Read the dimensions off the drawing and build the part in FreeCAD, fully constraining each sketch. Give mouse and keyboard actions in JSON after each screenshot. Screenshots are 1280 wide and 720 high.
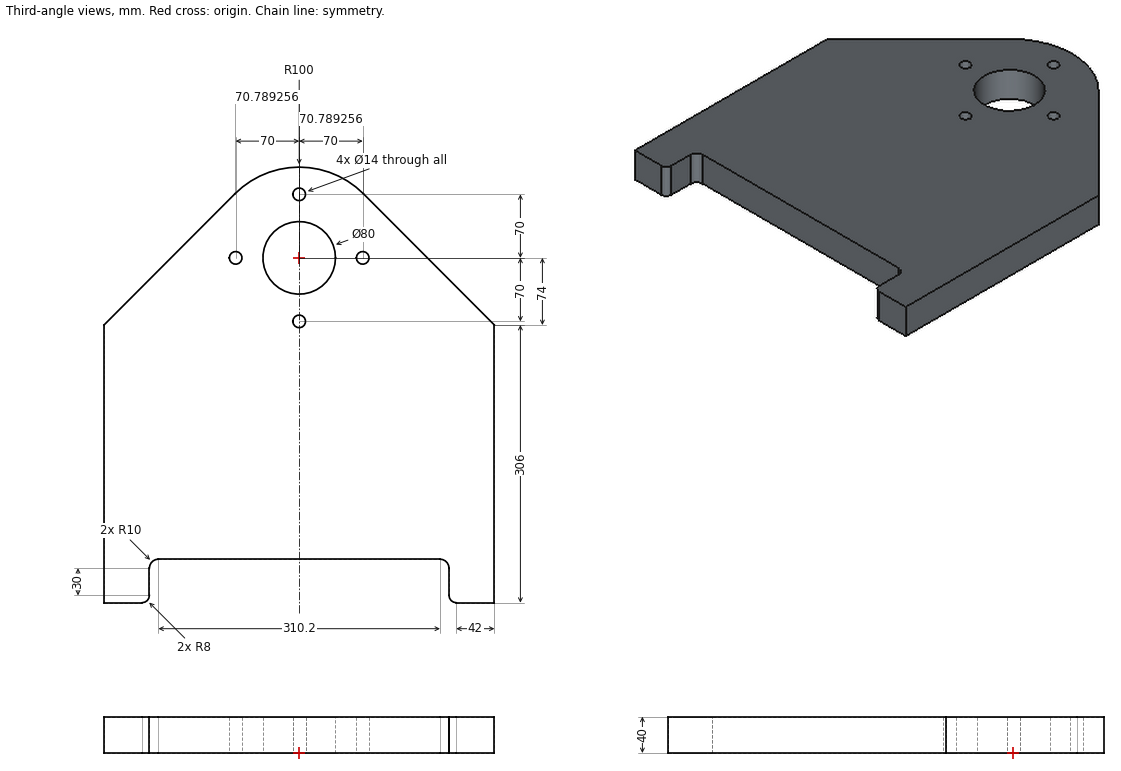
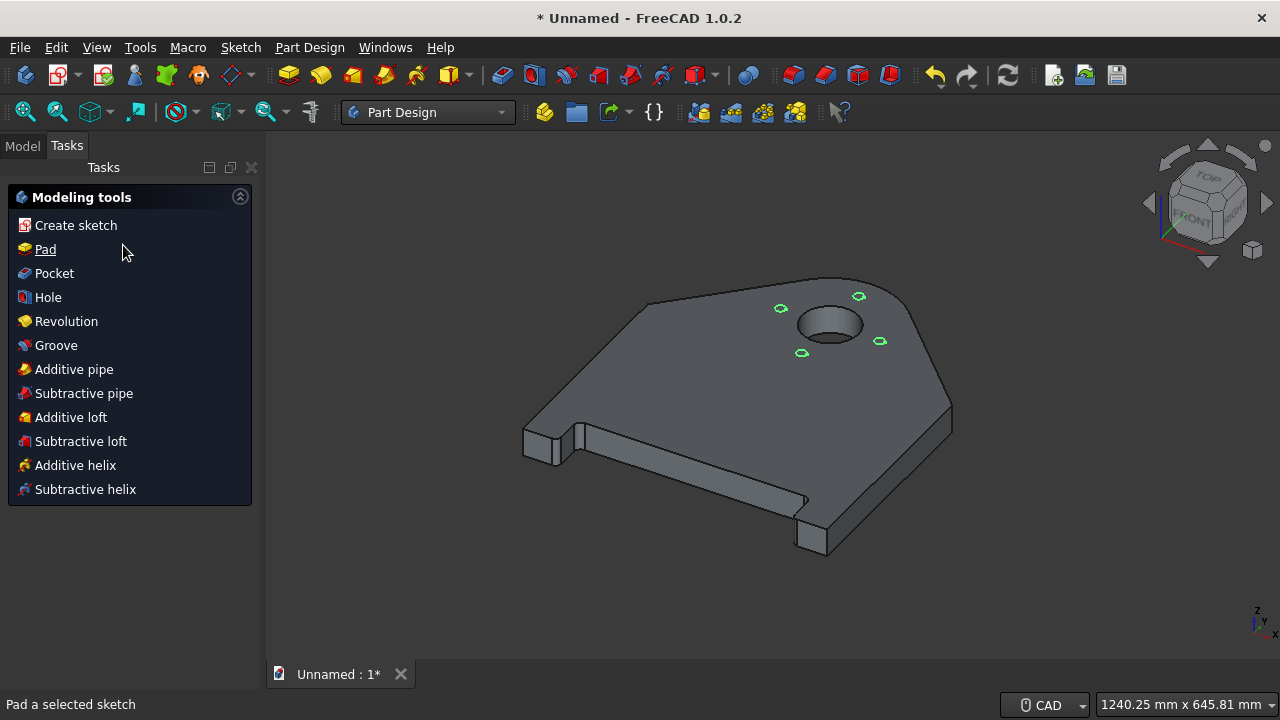
{"action": "left_click", "coordinate": [536, 76]}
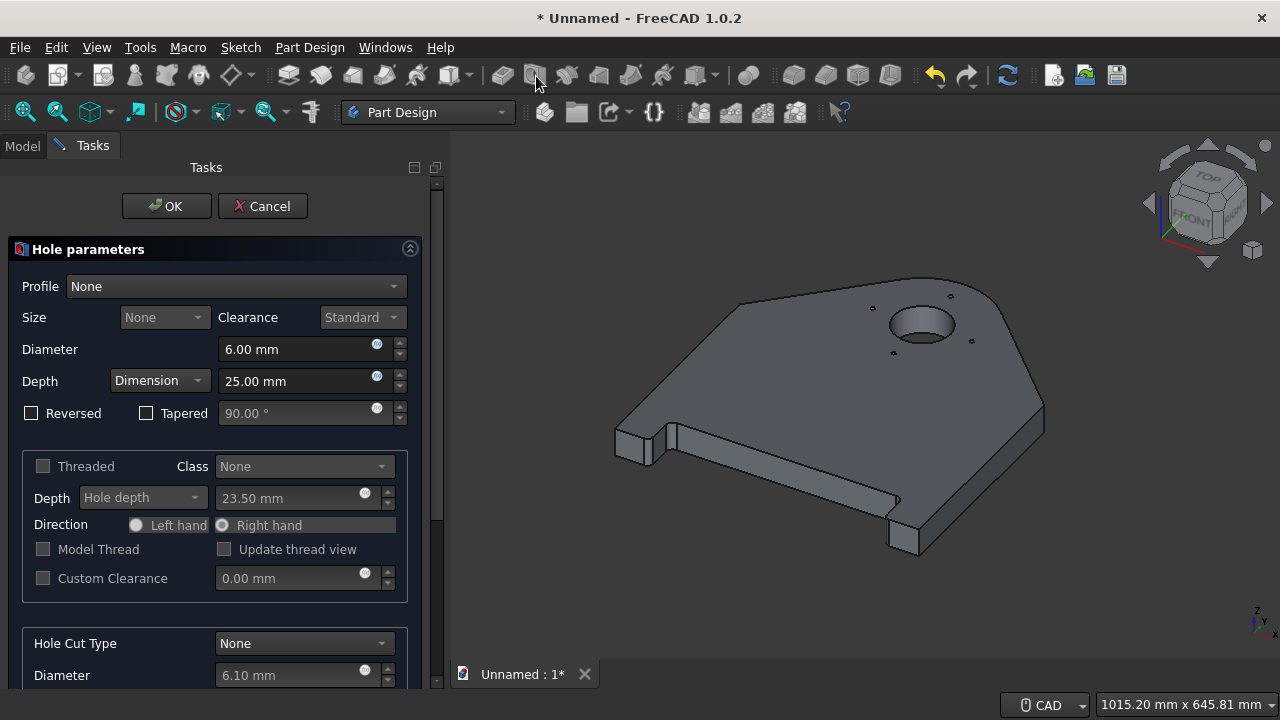
{"action": "triple_click", "coordinate": [305, 349]}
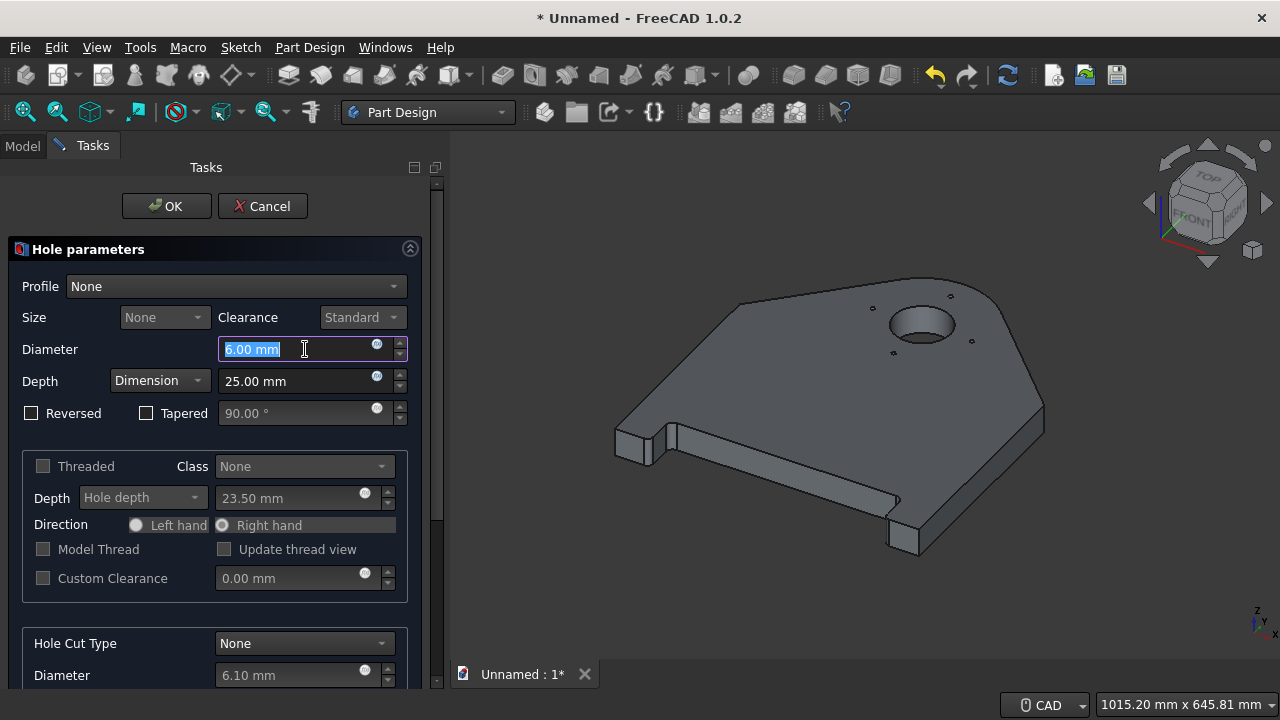
{"action": "type", "text": "14"}
{"action": "key", "text": "Tab"}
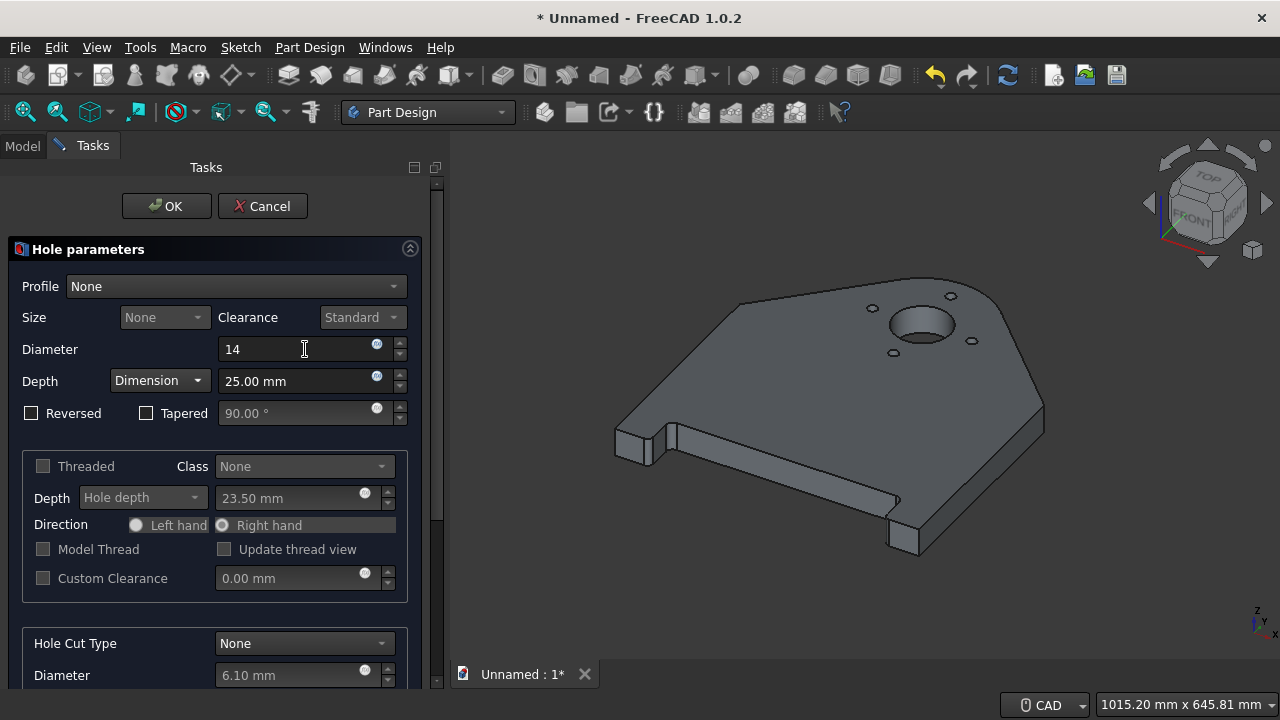
{"action": "left_click", "coordinate": [161, 380]}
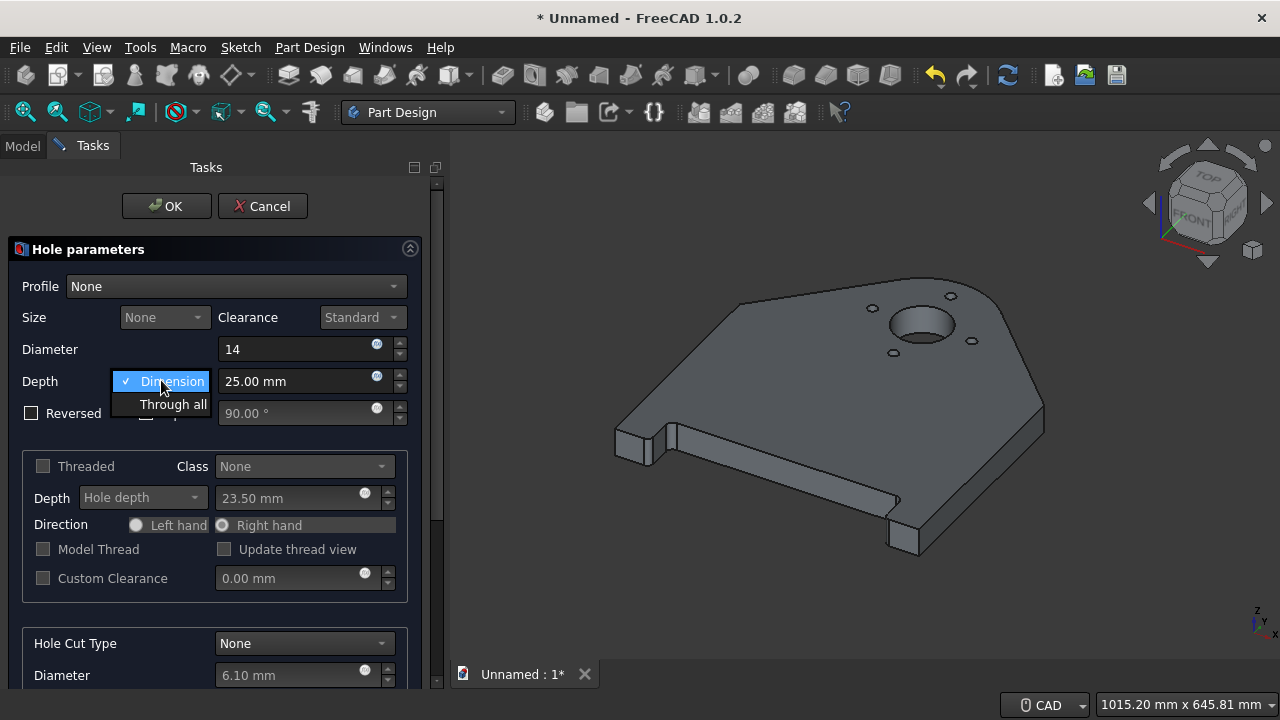
{"action": "left_click", "coordinate": [160, 404]}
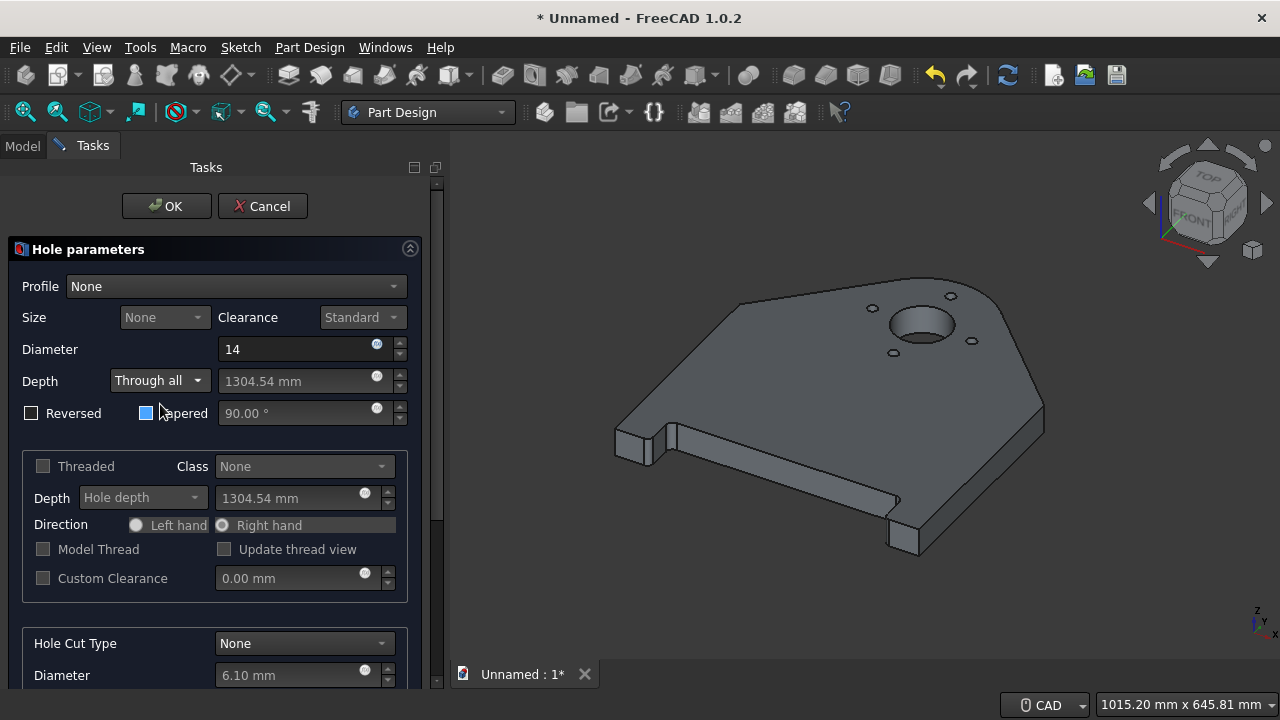
{"action": "left_click", "coordinate": [167, 206]}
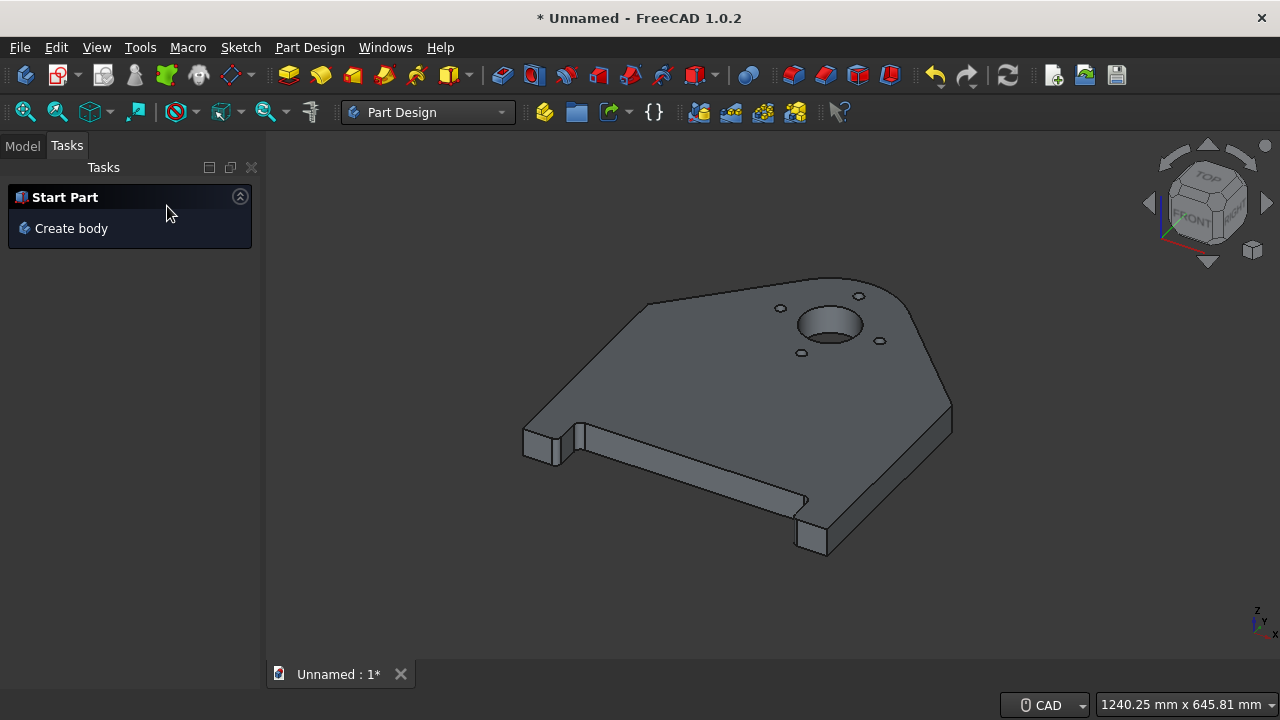
{"action": "key", "text": "0"}